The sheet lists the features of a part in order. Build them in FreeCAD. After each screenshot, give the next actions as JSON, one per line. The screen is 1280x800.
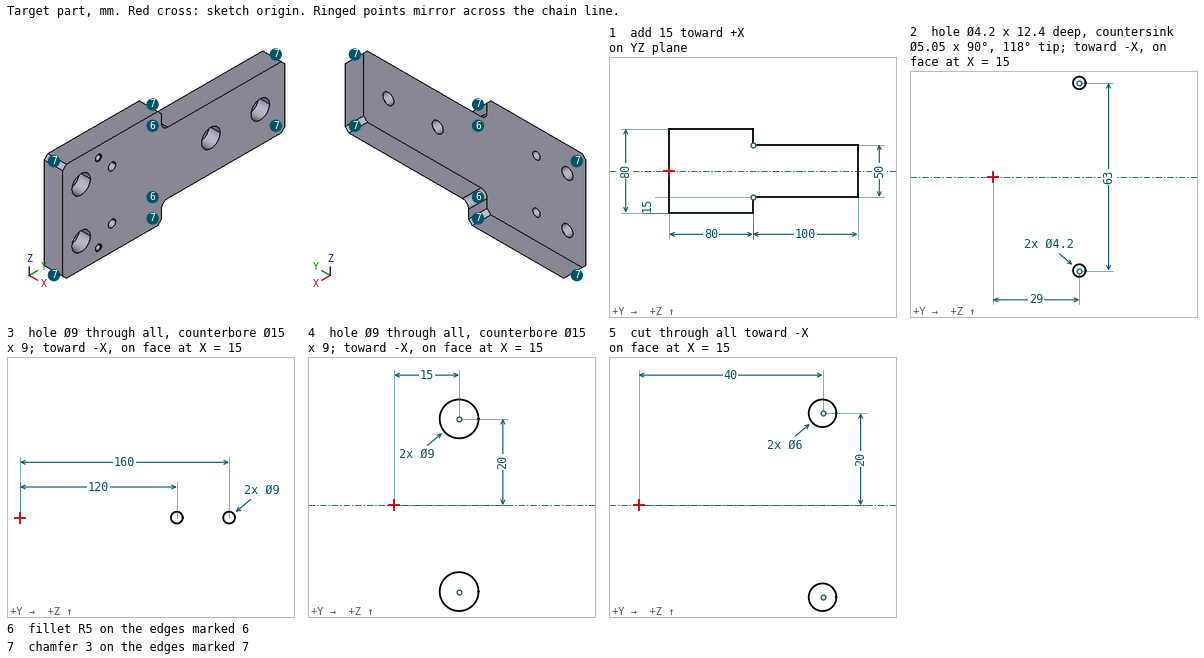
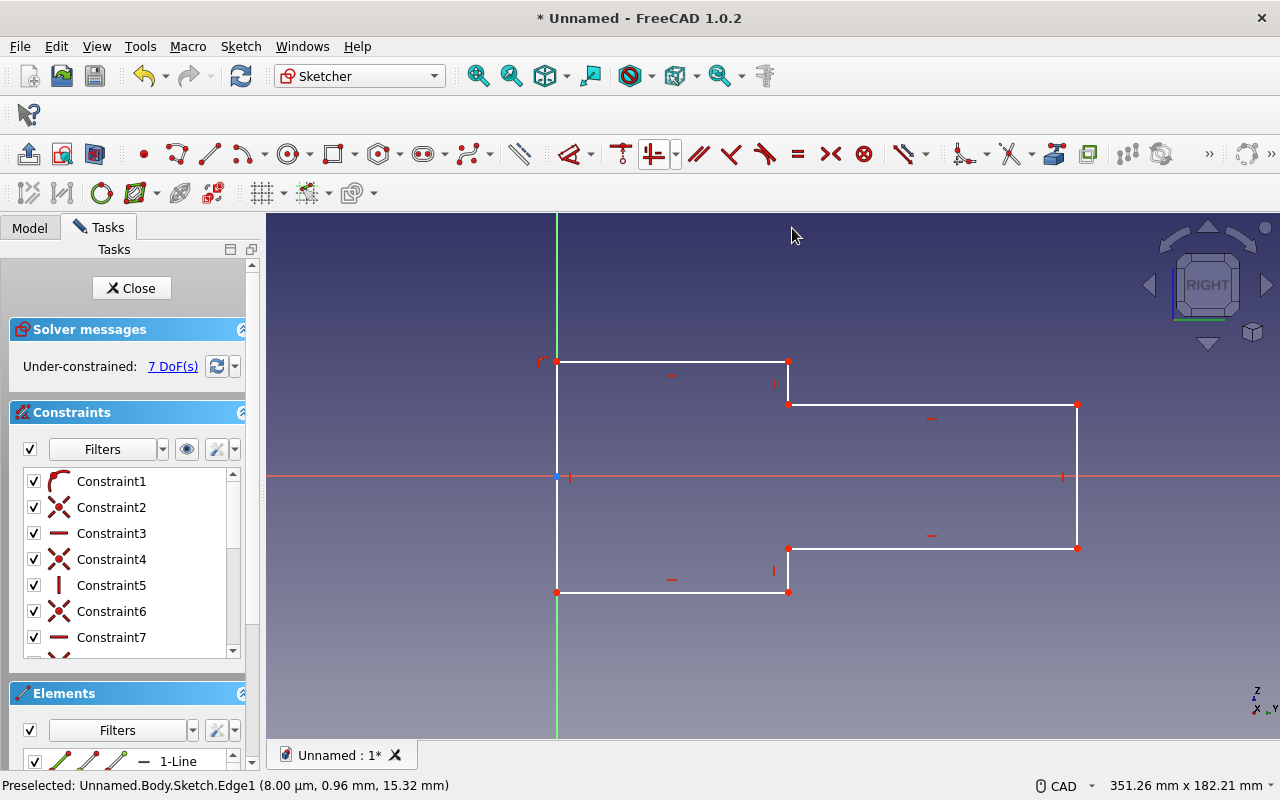
{"action": "left_click", "coordinate": [788, 549]}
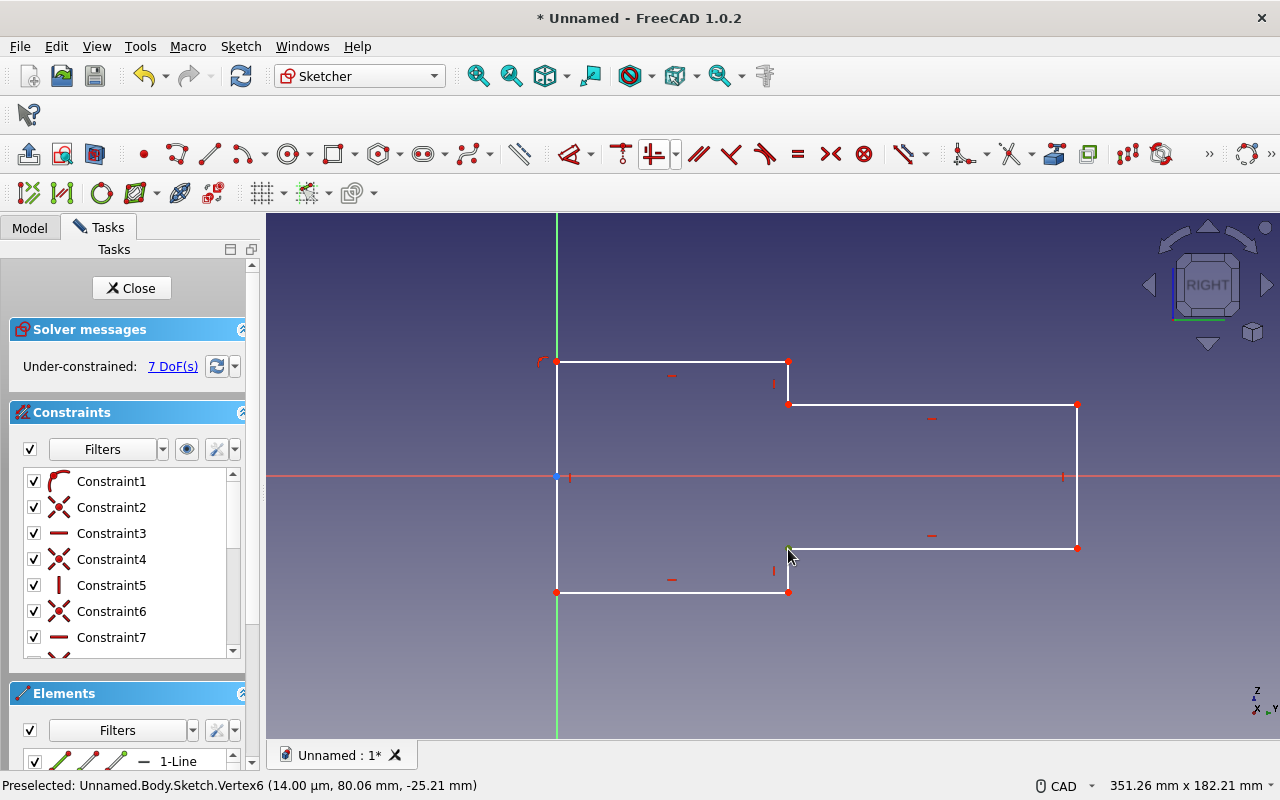
{"action": "left_click", "coordinate": [788, 405]}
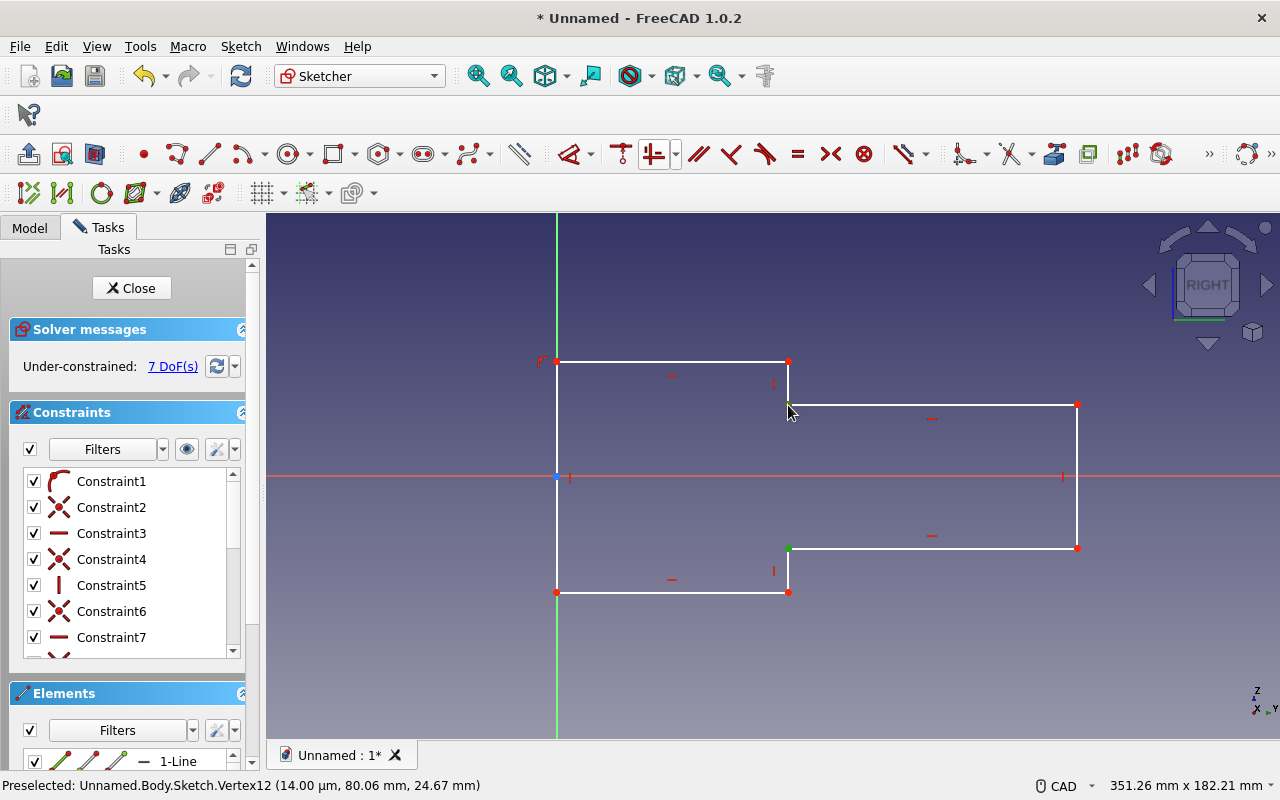
{"action": "left_click", "coordinate": [353, 476]}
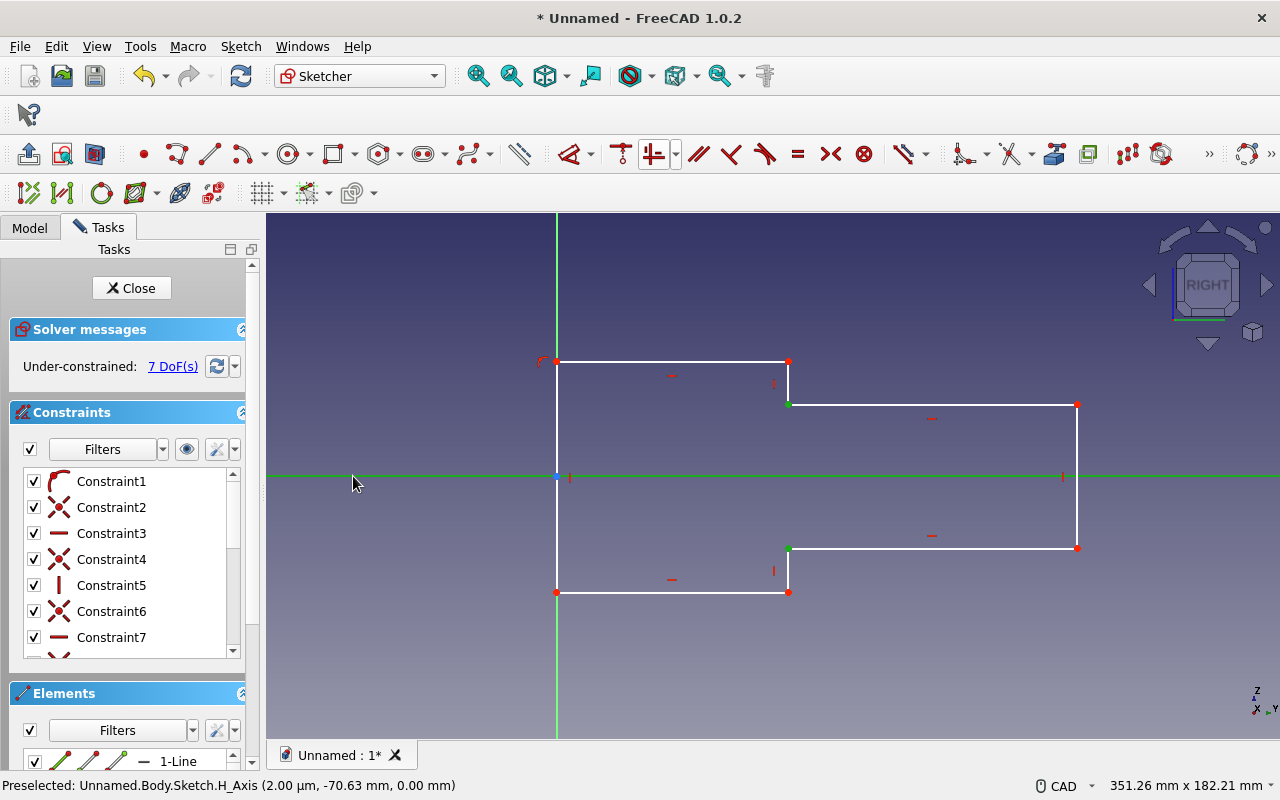
{"action": "left_click", "coordinate": [831, 154]}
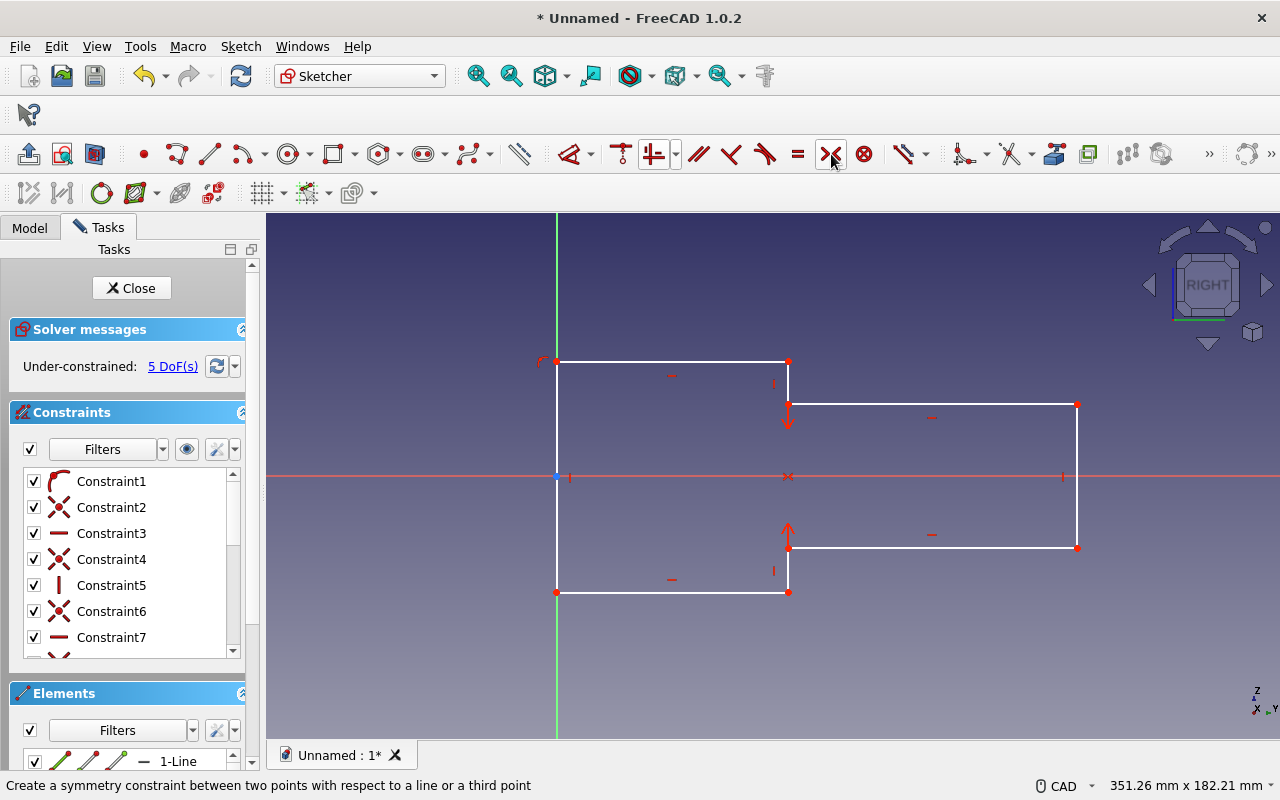
{"action": "key", "text": "d"}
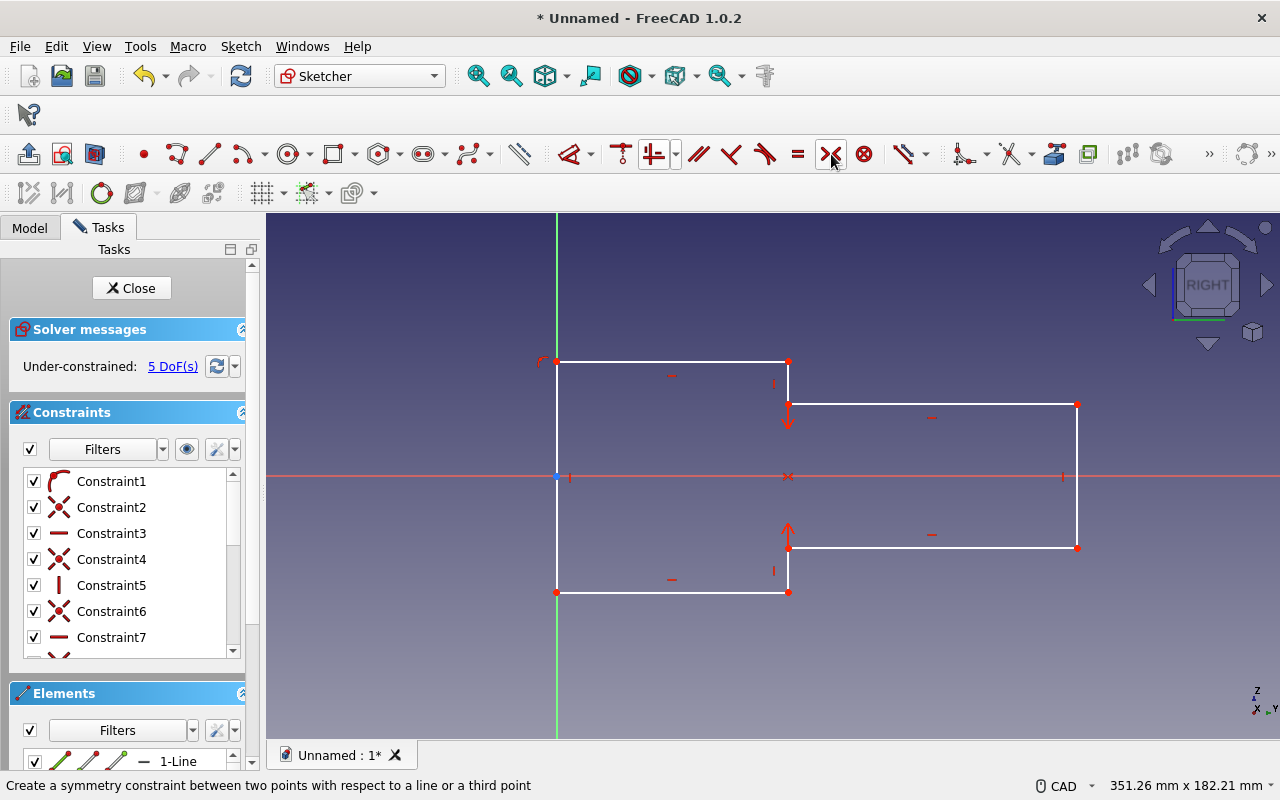
{"action": "left_click", "coordinate": [557, 431]}
{"action": "left_click", "coordinate": [523, 424]}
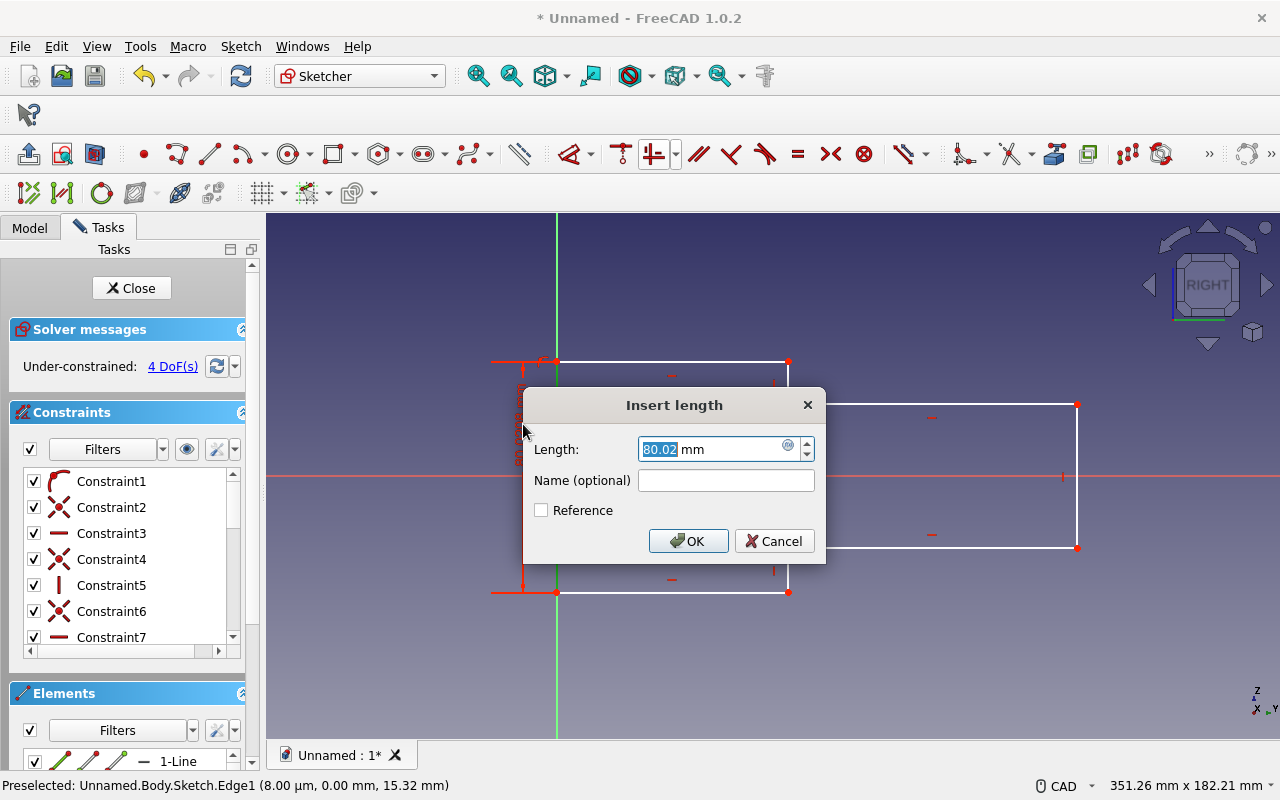
{"action": "type", "text": "80"}
{"action": "key", "text": "Return"}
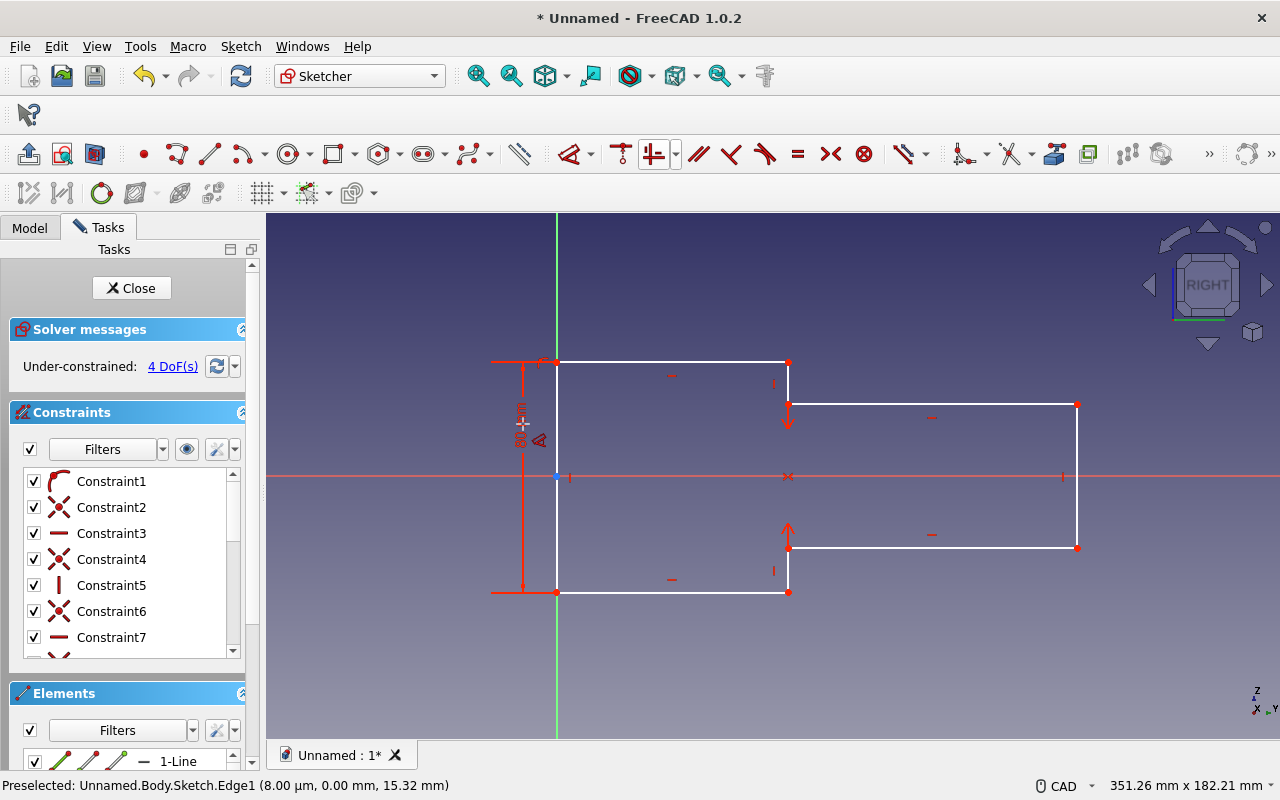
{"action": "left_click", "coordinate": [626, 593]}
{"action": "left_click", "coordinate": [672, 627]}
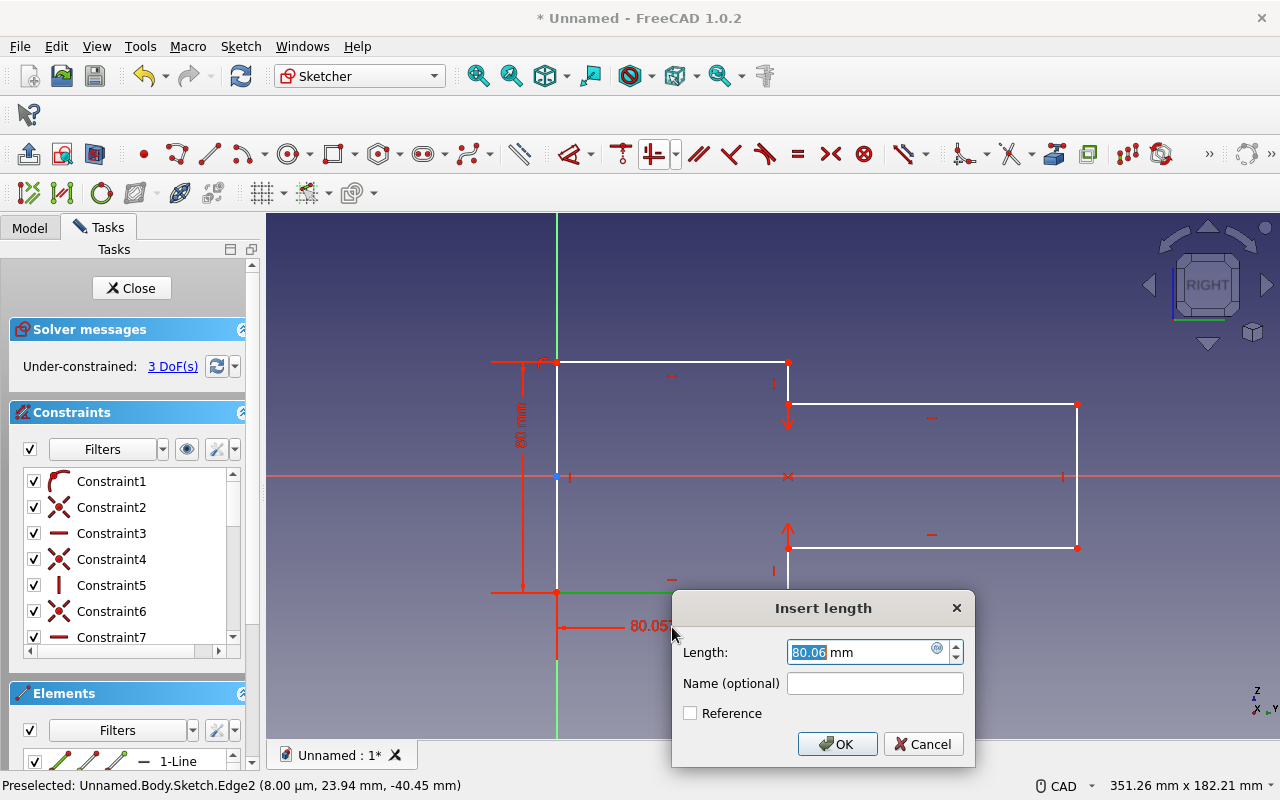
{"action": "type", "text": "80"}
{"action": "key", "text": "Return"}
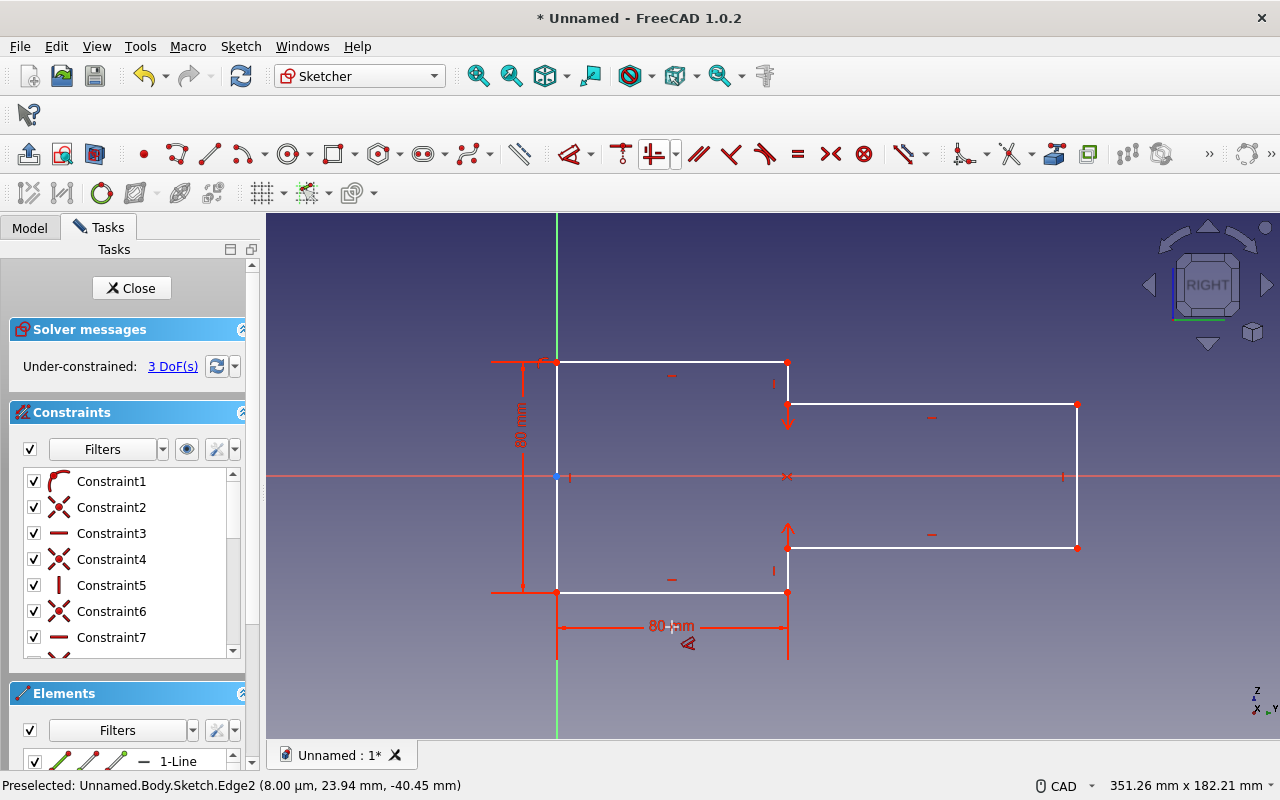
{"action": "left_click", "coordinate": [788, 580]}
{"action": "left_click", "coordinate": [754, 571]}